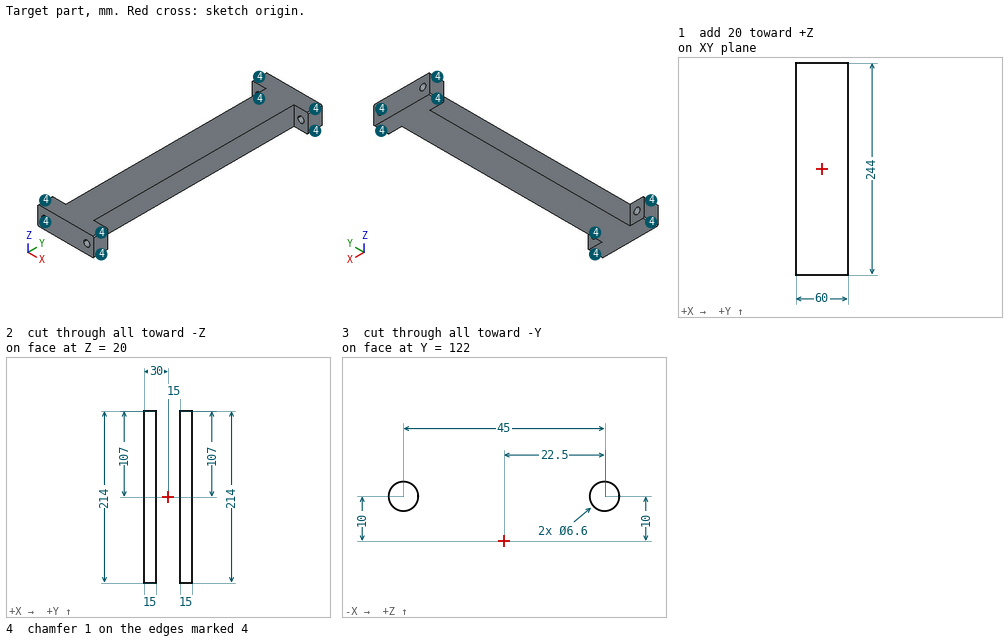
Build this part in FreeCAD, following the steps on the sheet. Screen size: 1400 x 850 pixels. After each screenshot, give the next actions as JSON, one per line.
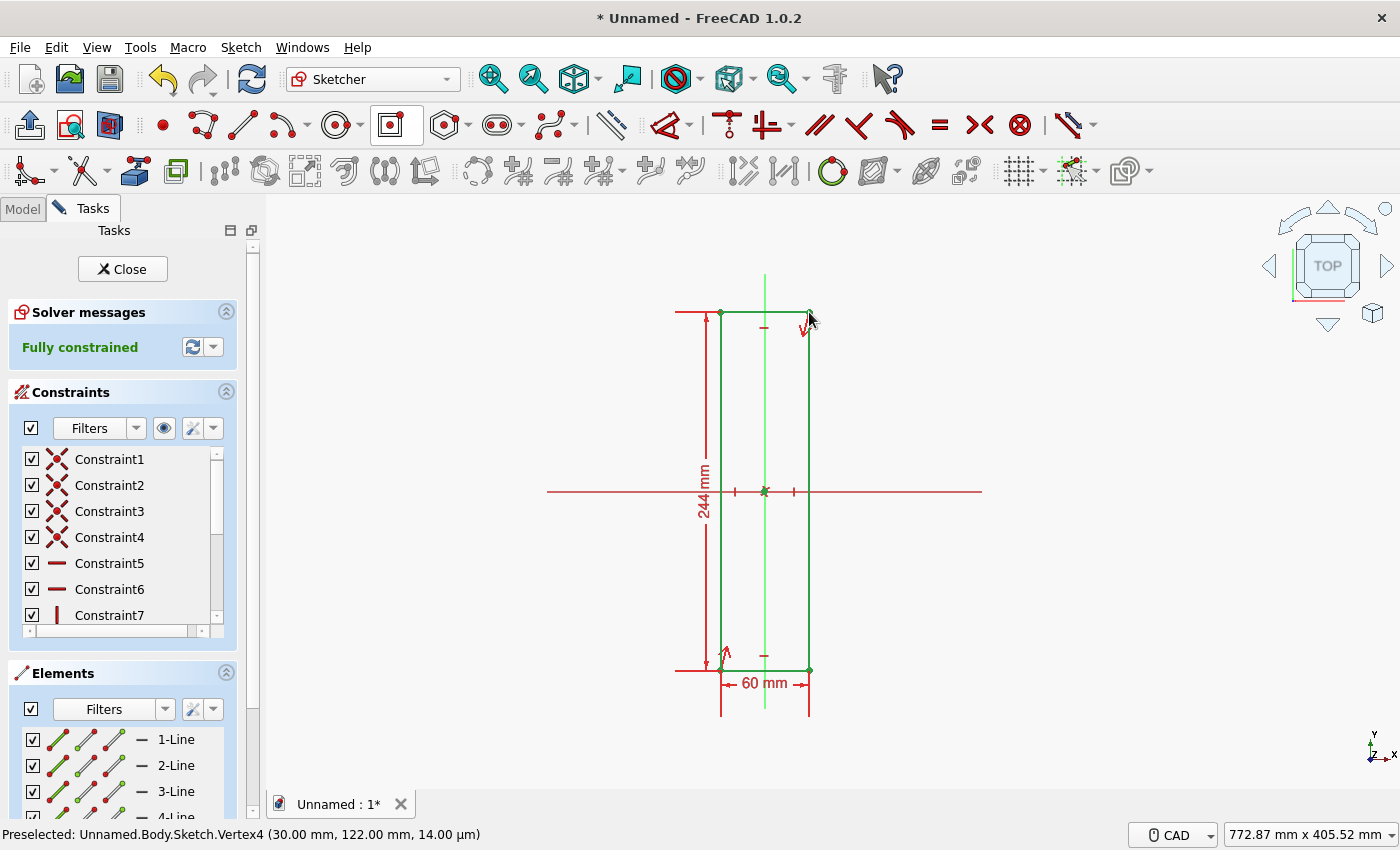
{"action": "left_click", "coordinate": [123, 269]}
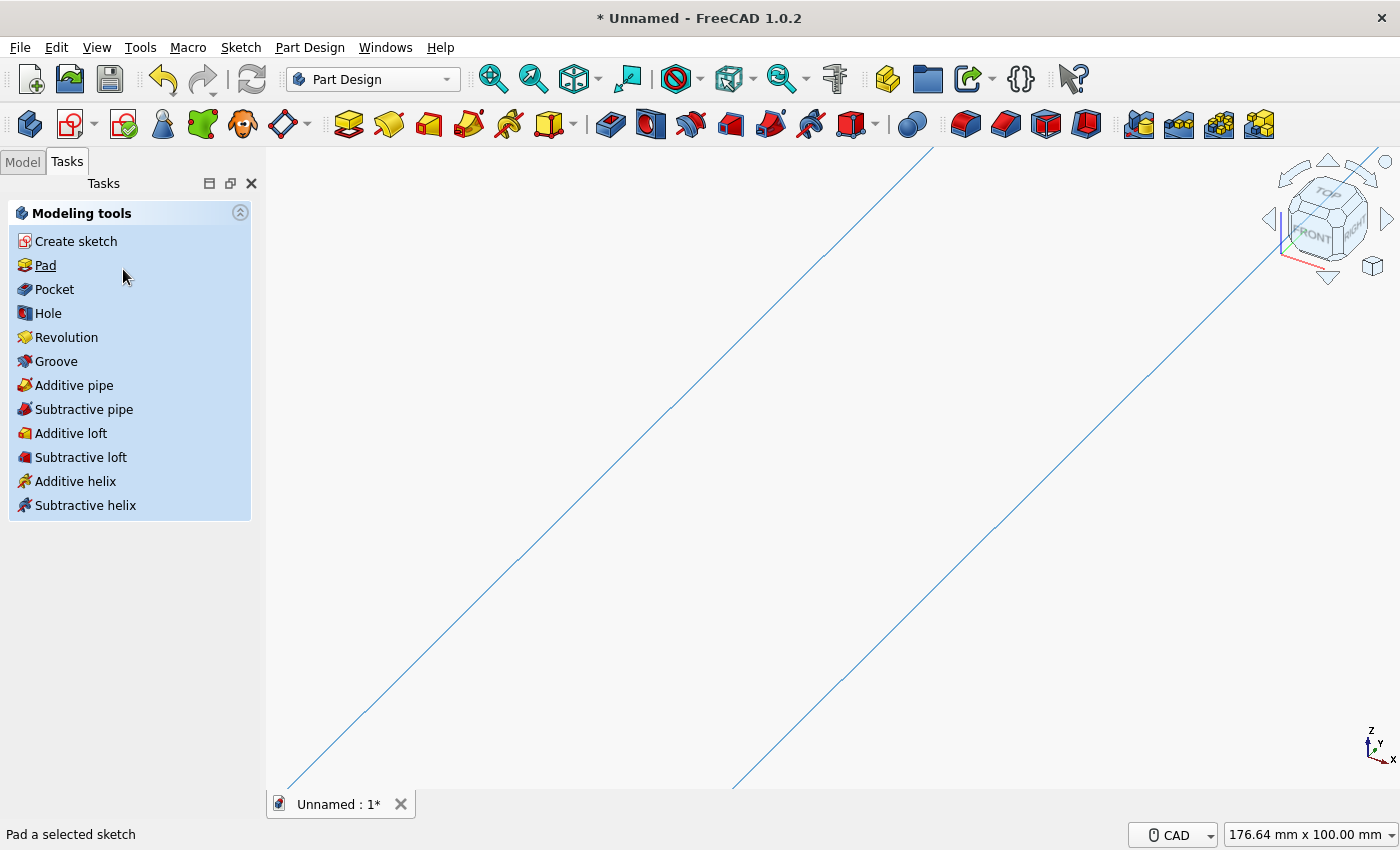
{"action": "left_click", "coordinate": [350, 124]}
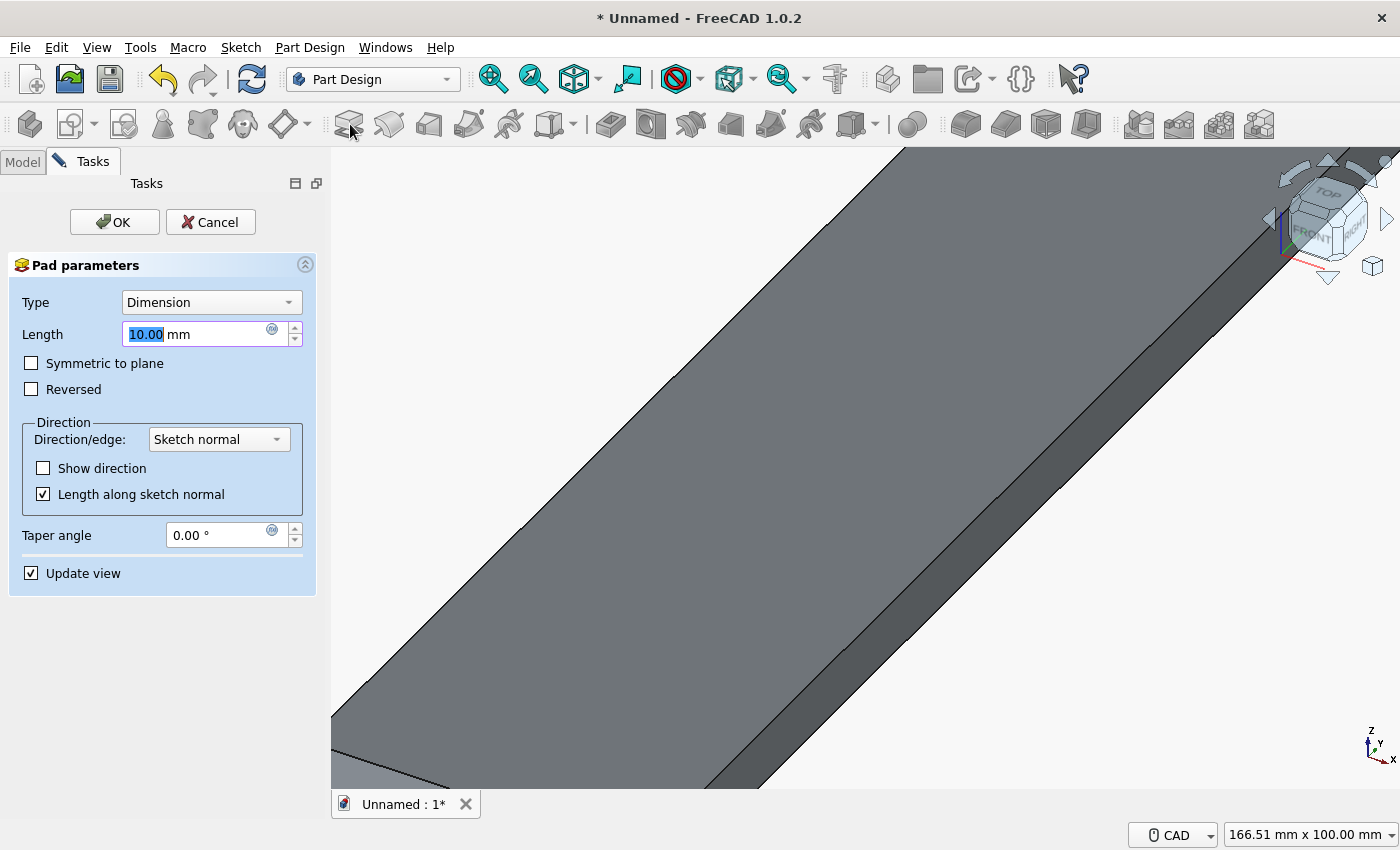
{"action": "type", "text": "20"}
{"action": "key", "text": "Tab"}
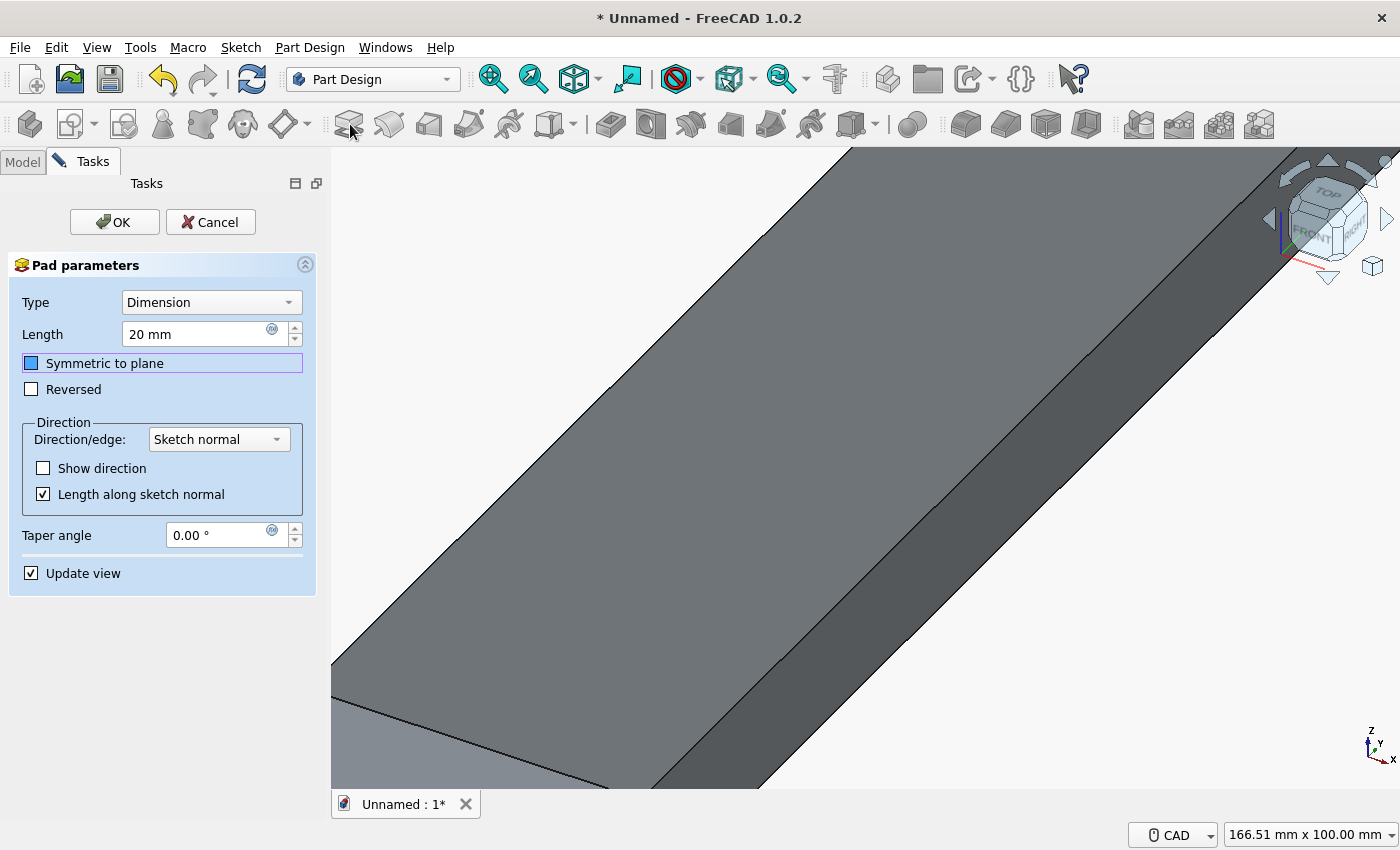
{"action": "left_click", "coordinate": [115, 222]}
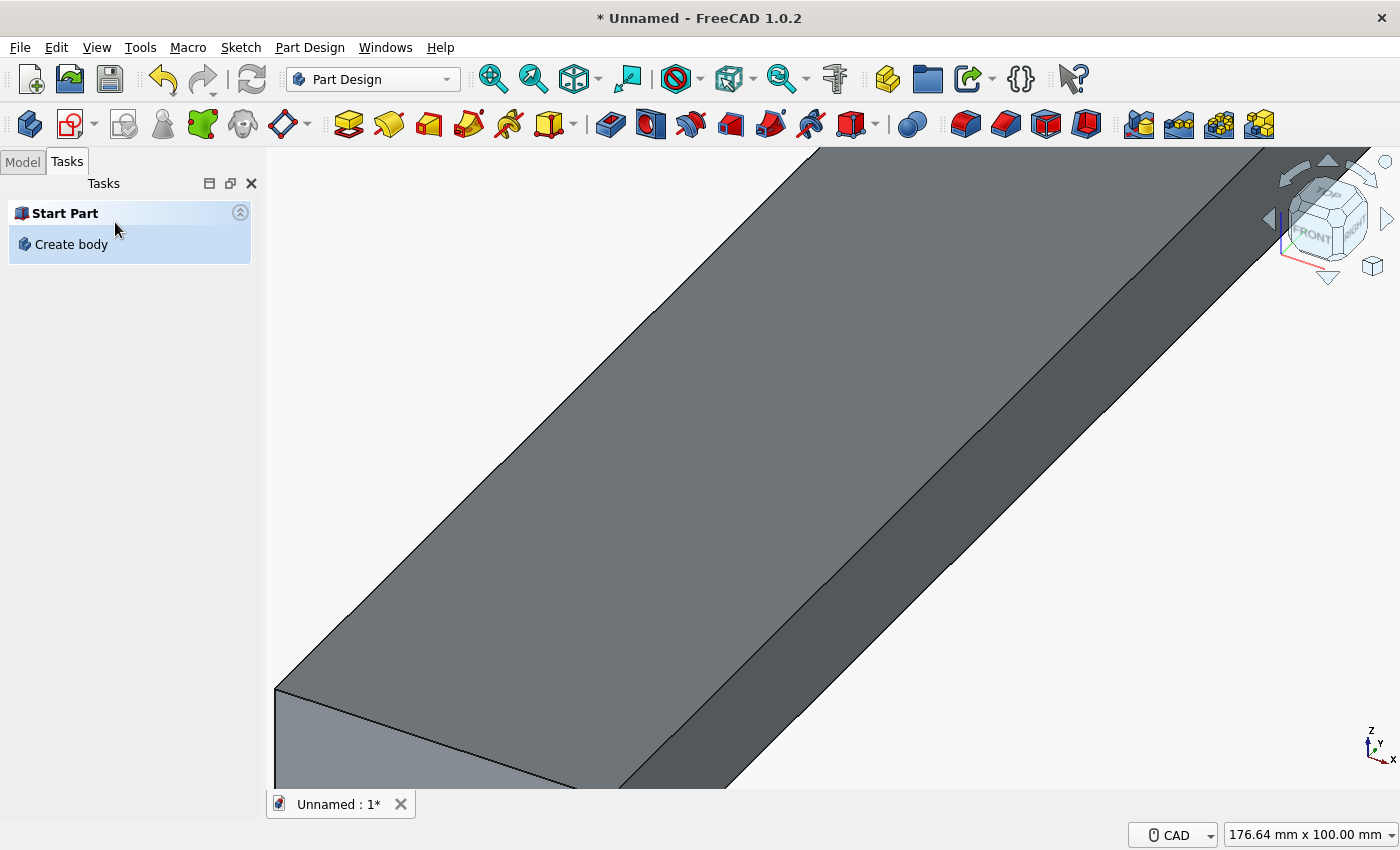
{"action": "left_click", "coordinate": [494, 80]}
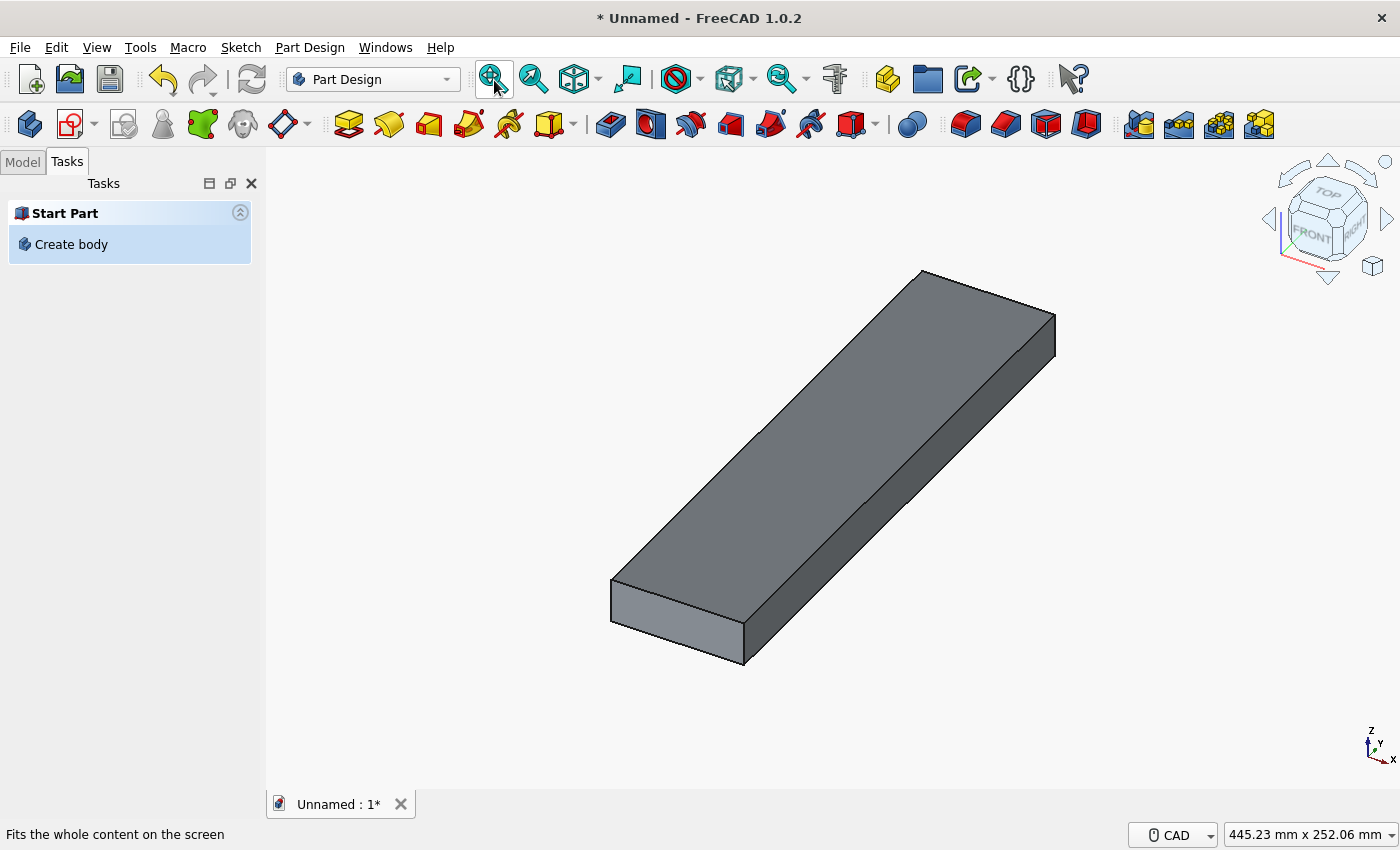
{"action": "left_click", "coordinate": [922, 358]}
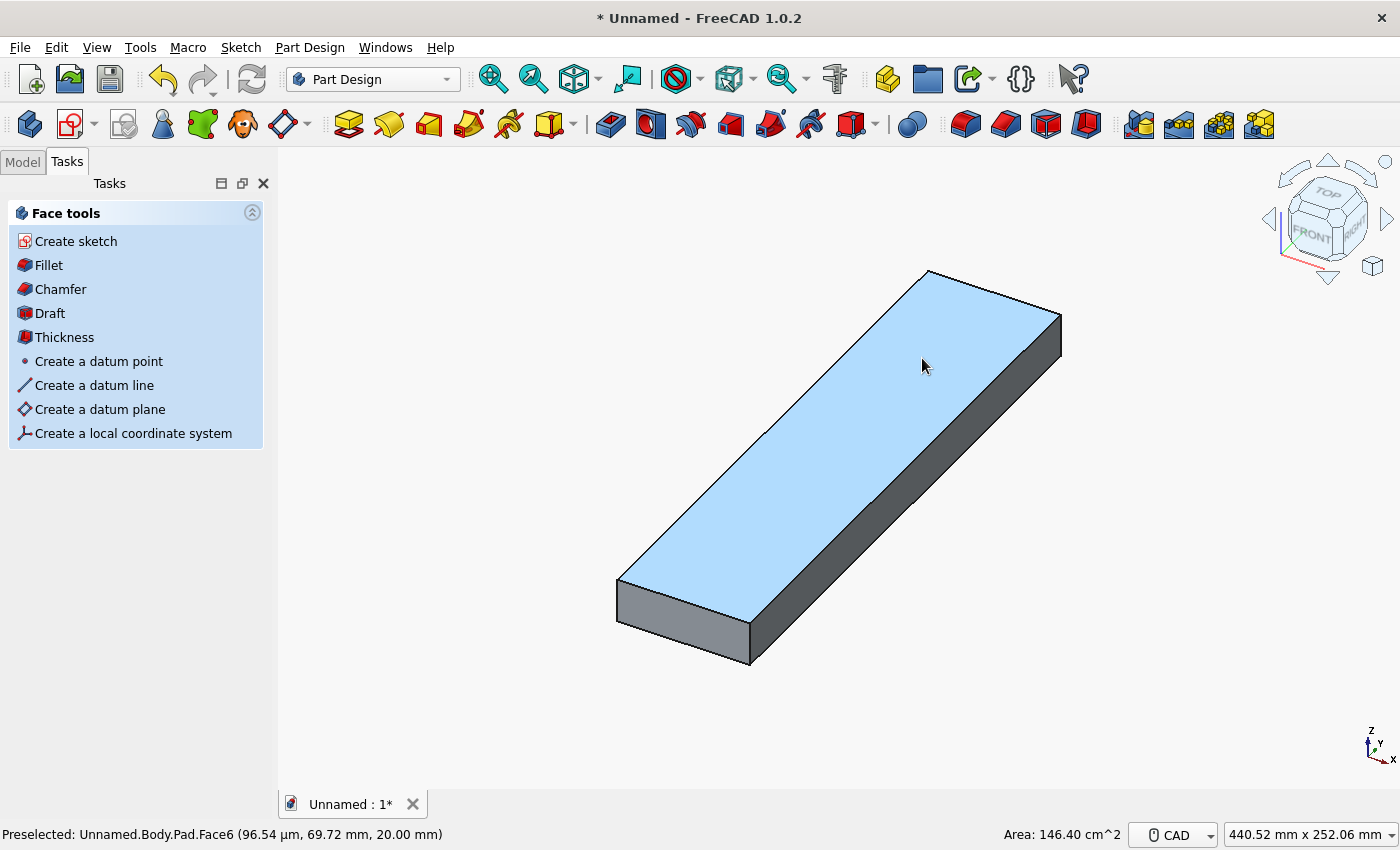
{"action": "left_click", "coordinate": [70, 124]}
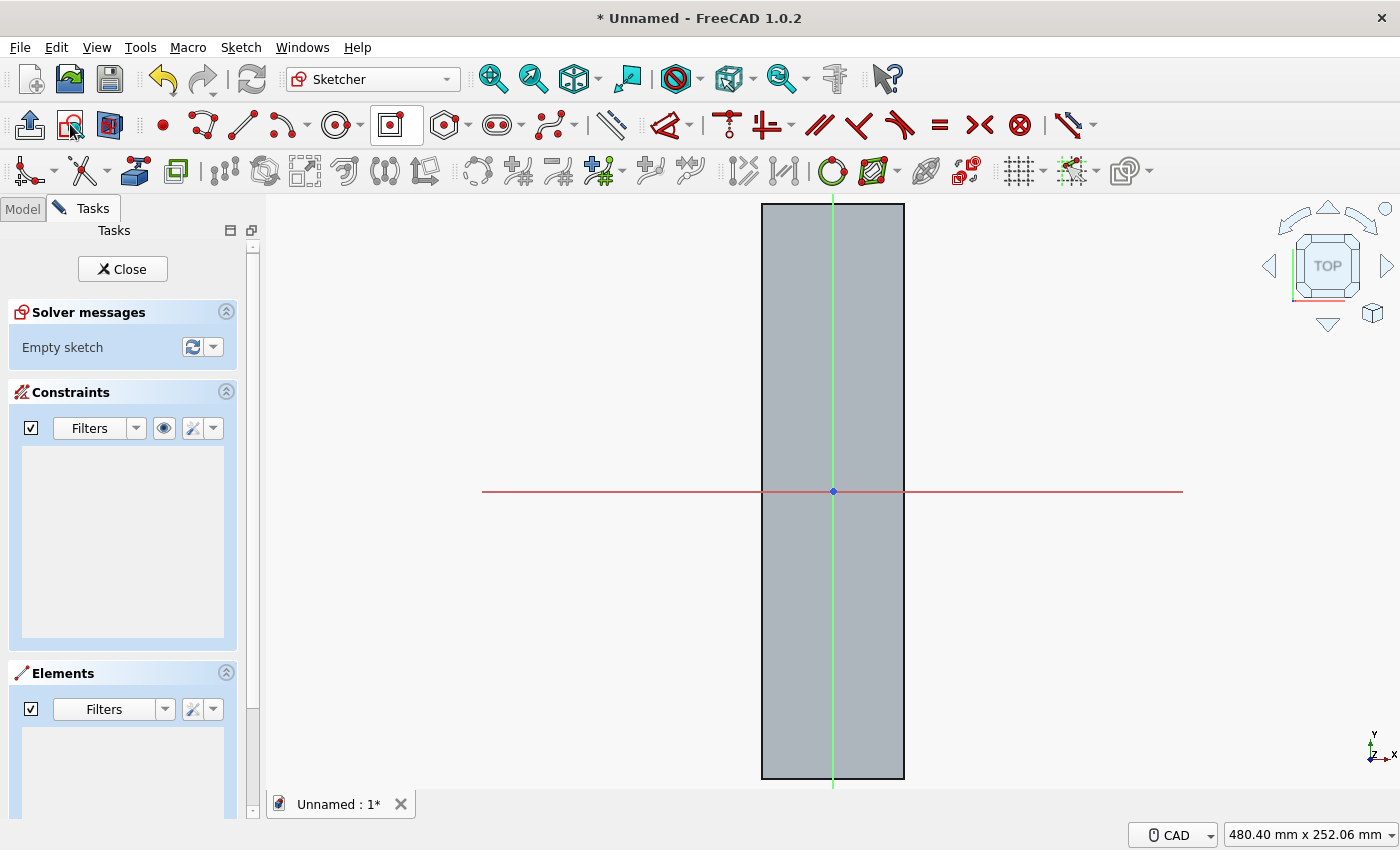
{"action": "scroll", "coordinate": [455, 492], "scroll_direction": "down", "scroll_amount": 1}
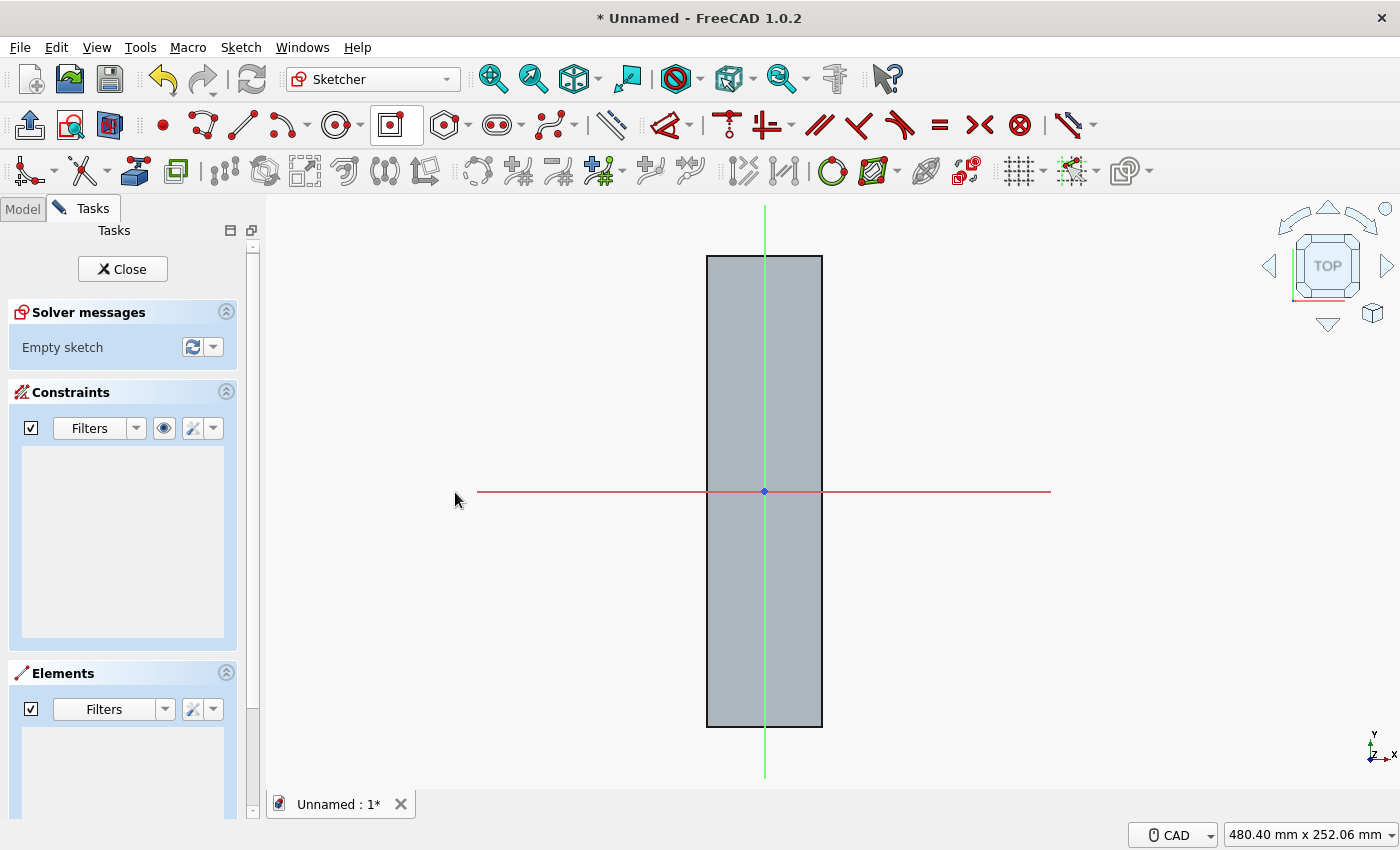
{"action": "left_click", "coordinate": [418, 126]}